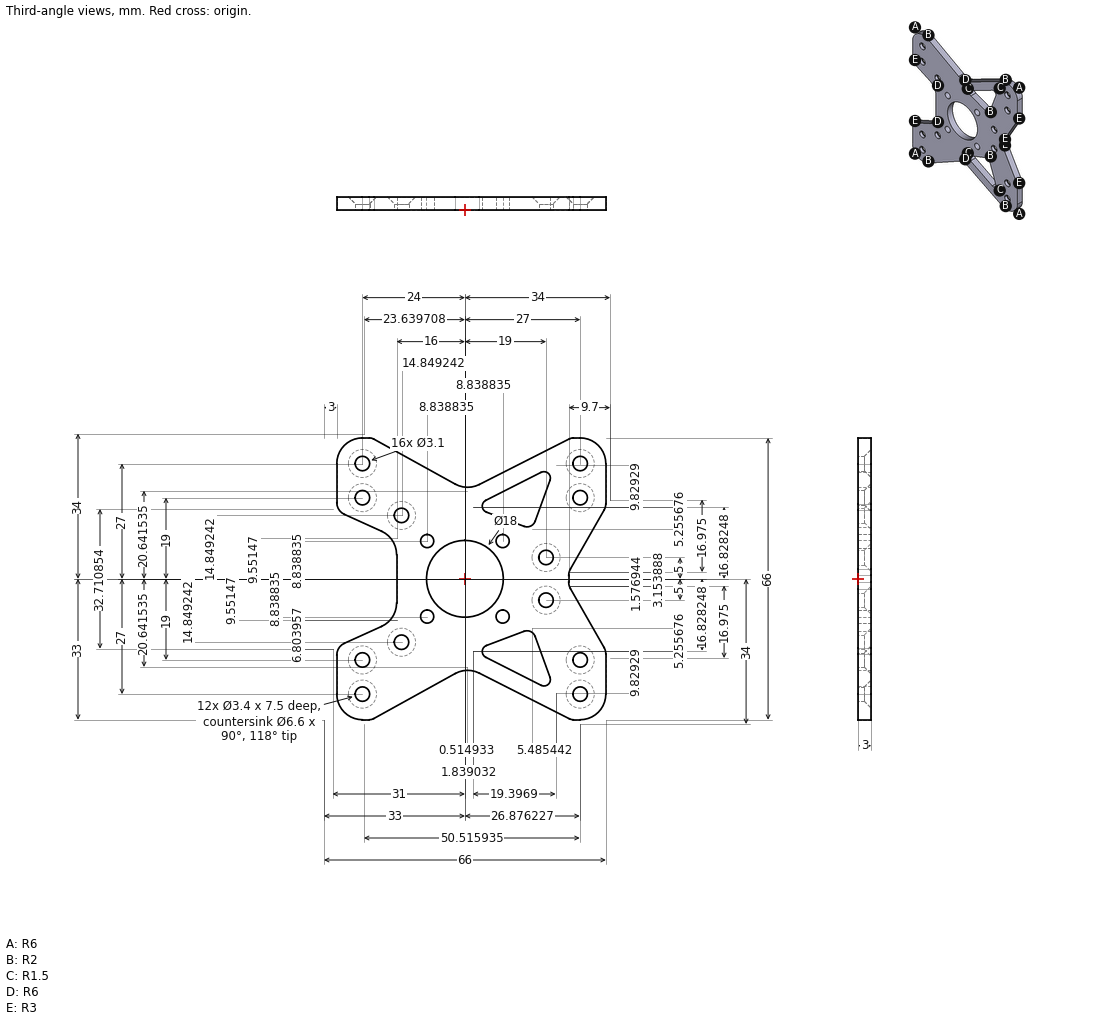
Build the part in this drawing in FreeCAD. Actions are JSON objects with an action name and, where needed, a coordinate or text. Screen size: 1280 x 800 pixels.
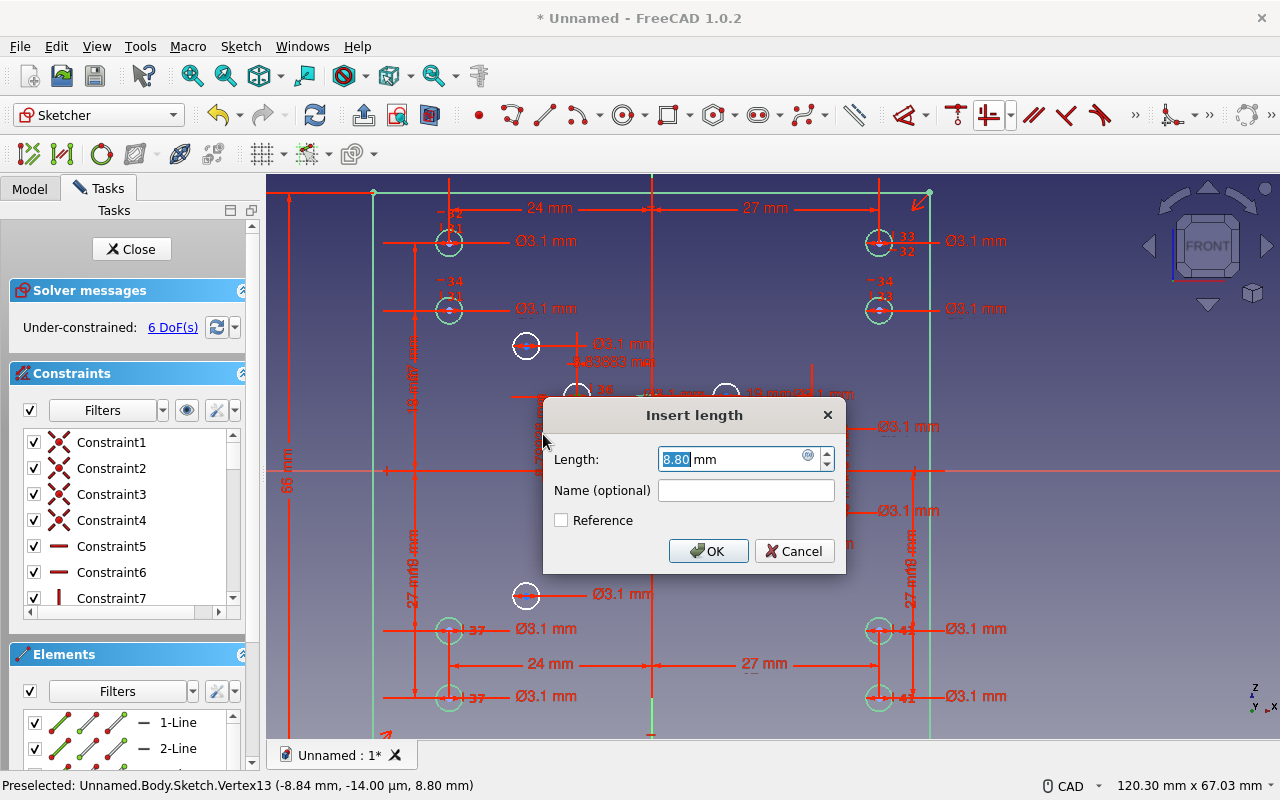
{"action": "type", "text": "8.838835"}
{"action": "key", "text": "Return"}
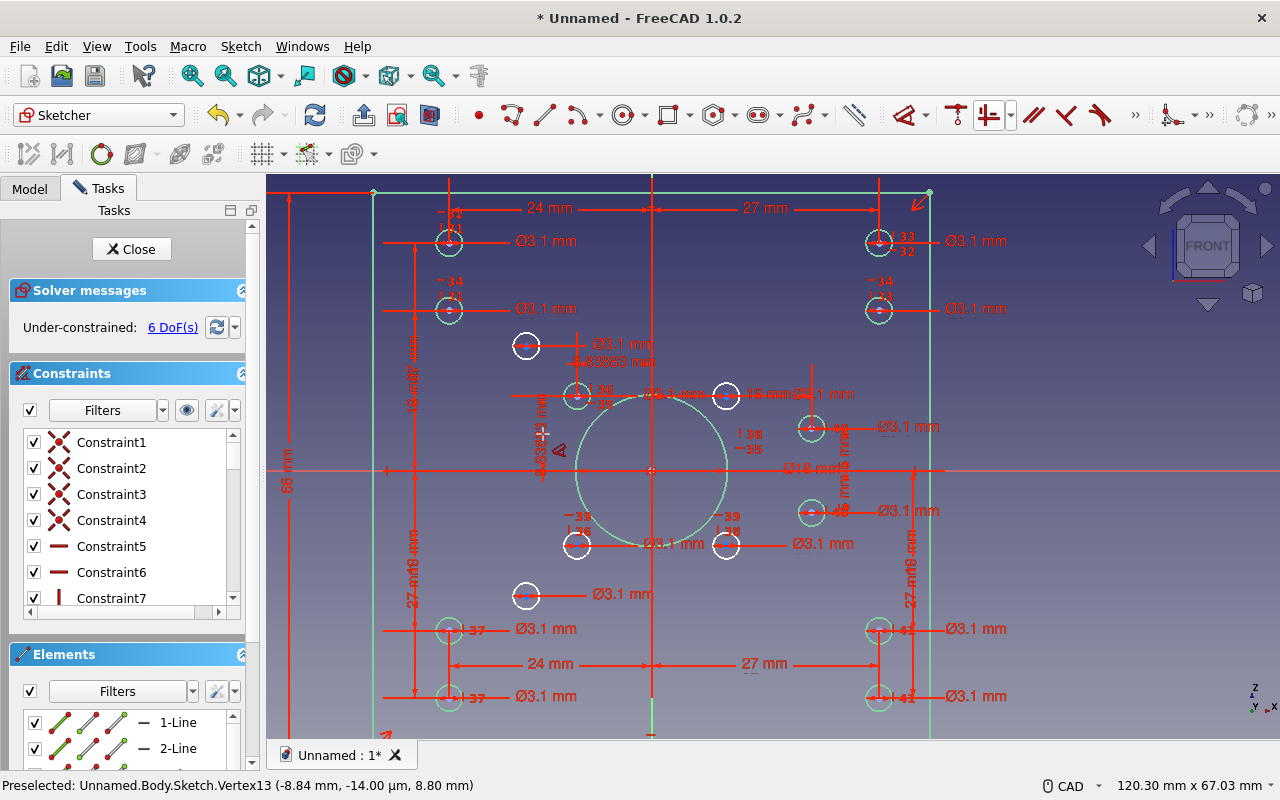
{"action": "left_click", "coordinate": [726, 396]}
{"action": "left_click", "coordinate": [689, 362]}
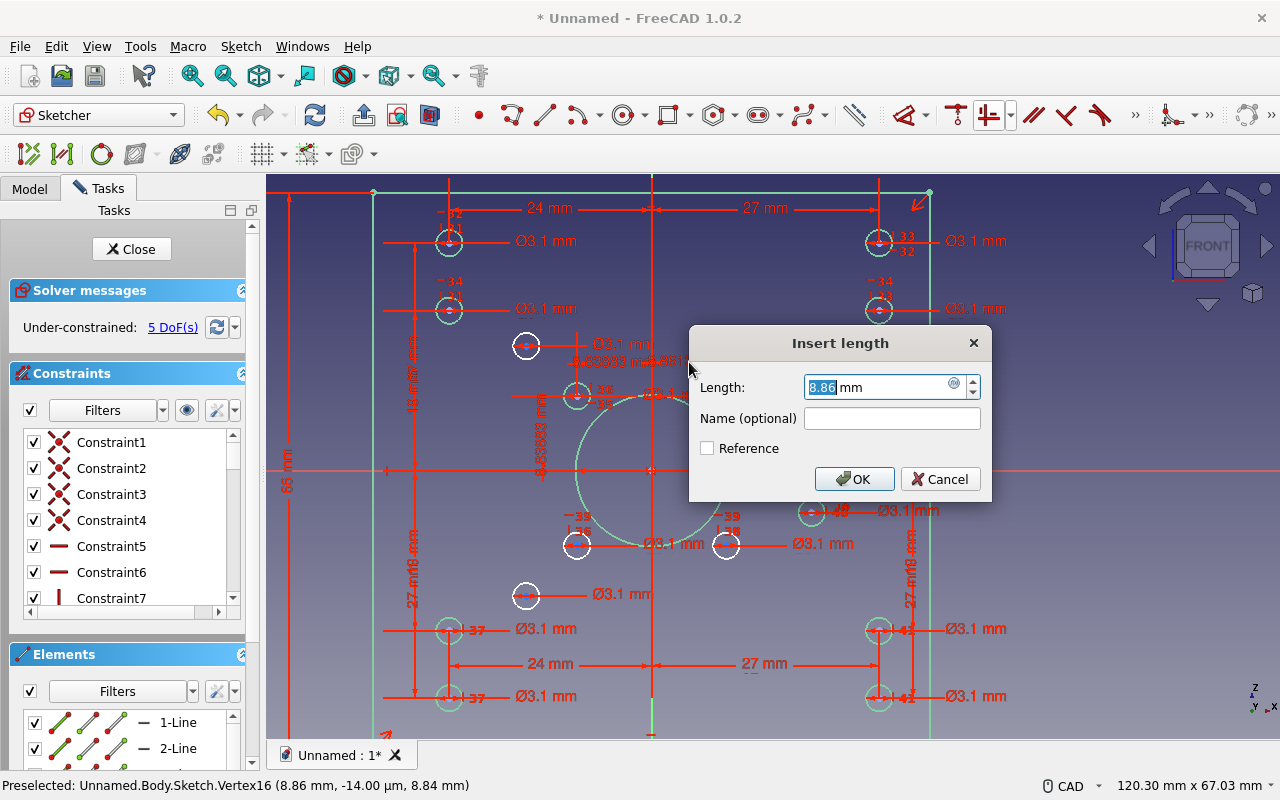
{"action": "type", "text": "8.838835"}
{"action": "key", "text": "Return"}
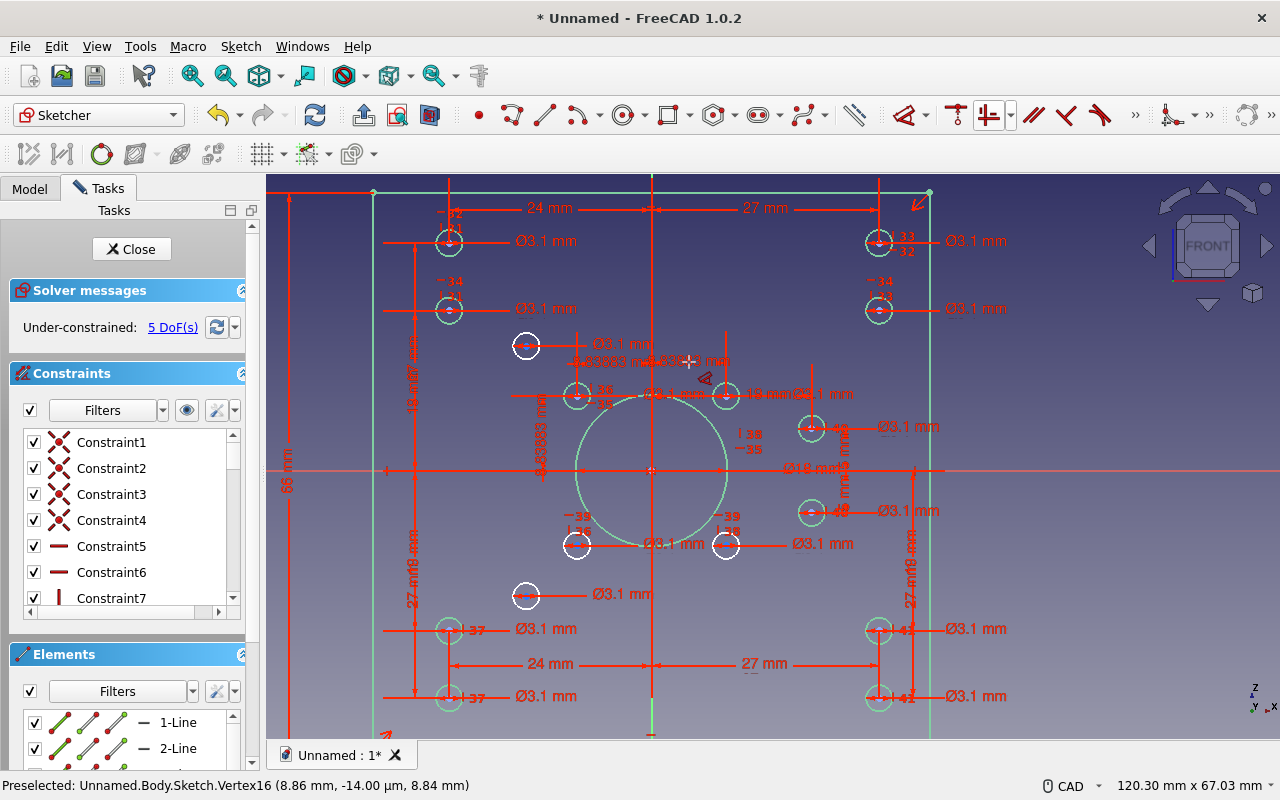
{"action": "left_click", "coordinate": [577, 546]}
{"action": "left_click", "coordinate": [543, 508]}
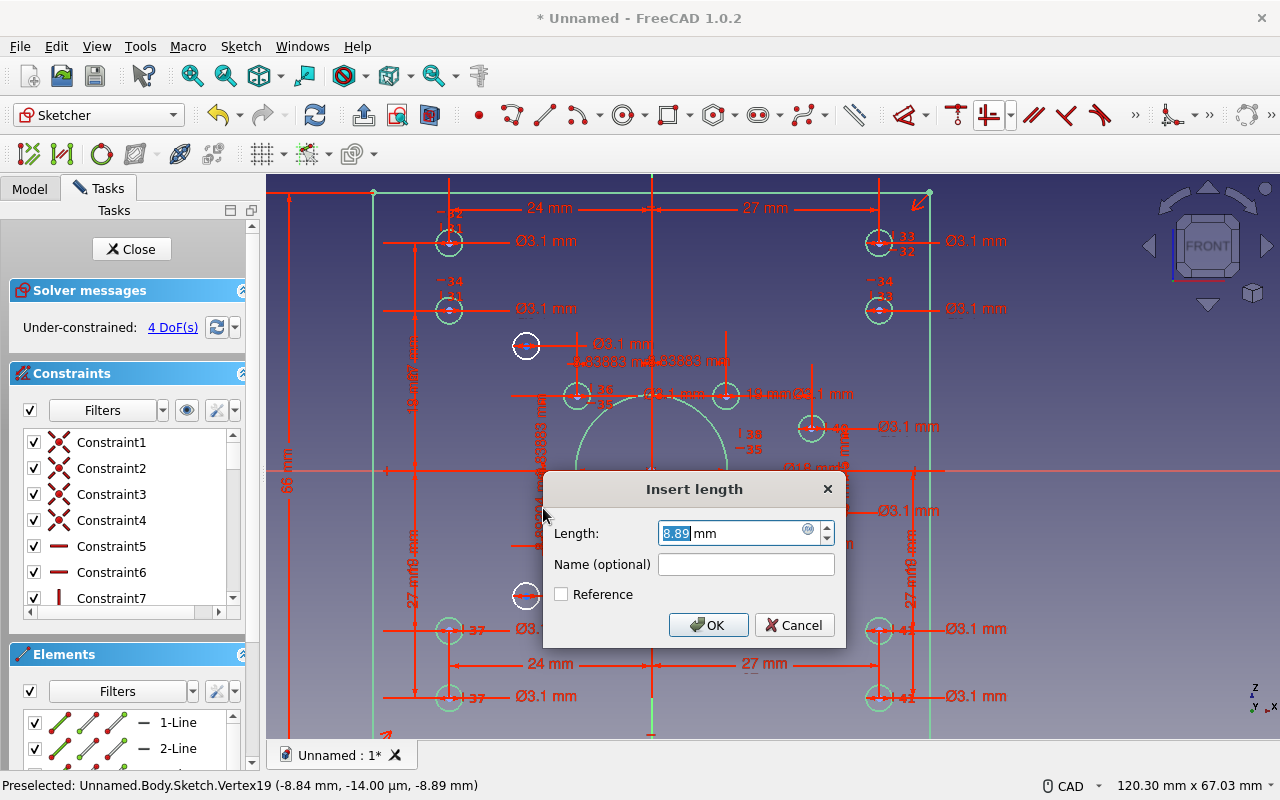
{"action": "type", "text": "8.838835"}
{"action": "key", "text": "Return"}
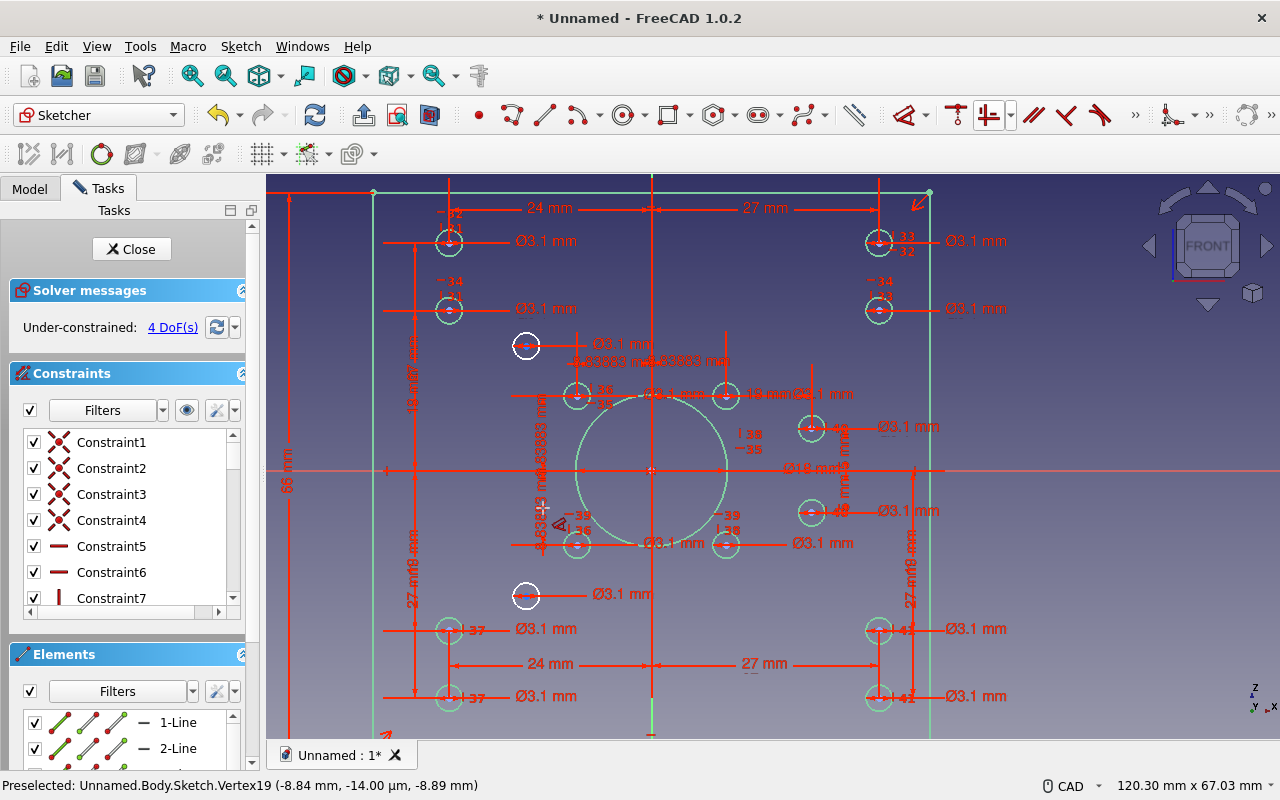
{"action": "left_click", "coordinate": [526, 346]}
{"action": "left_click", "coordinate": [589, 312]}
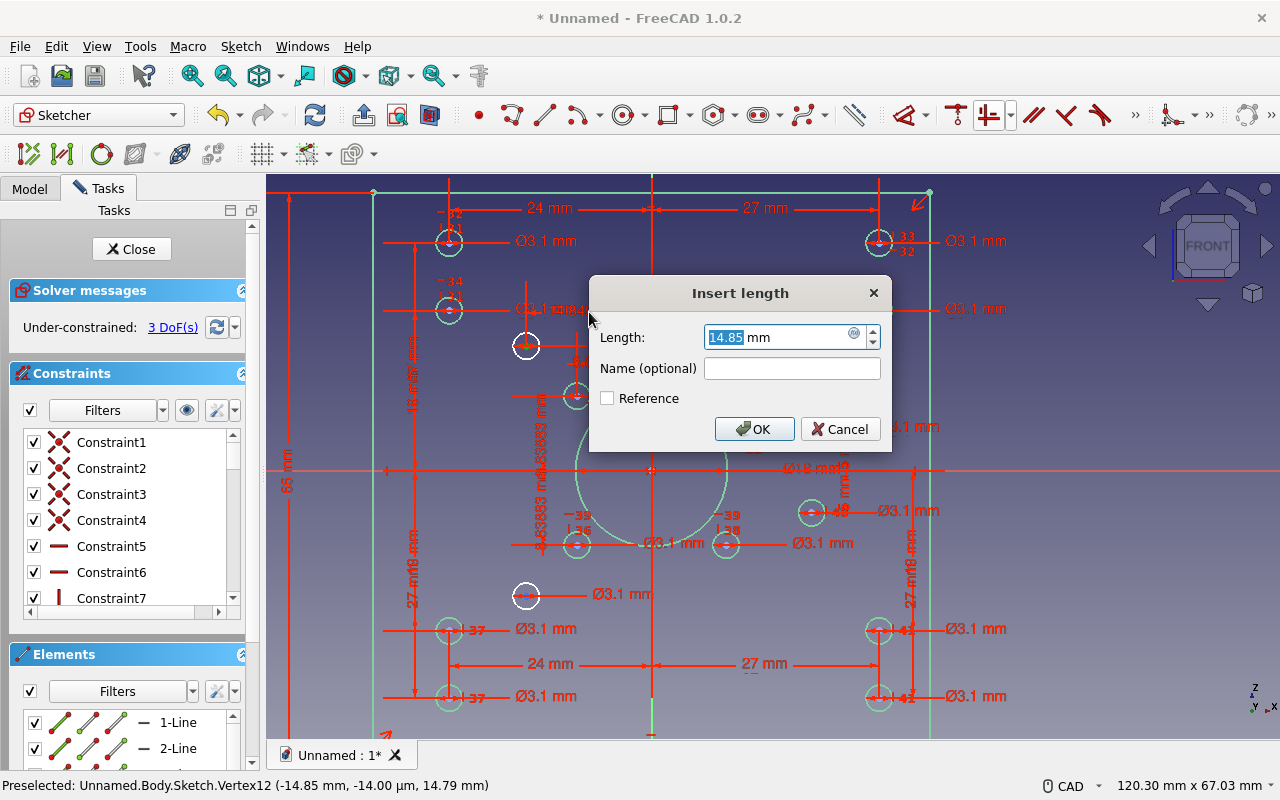
{"action": "type", "text": "14.849242"}
{"action": "key", "text": "Return"}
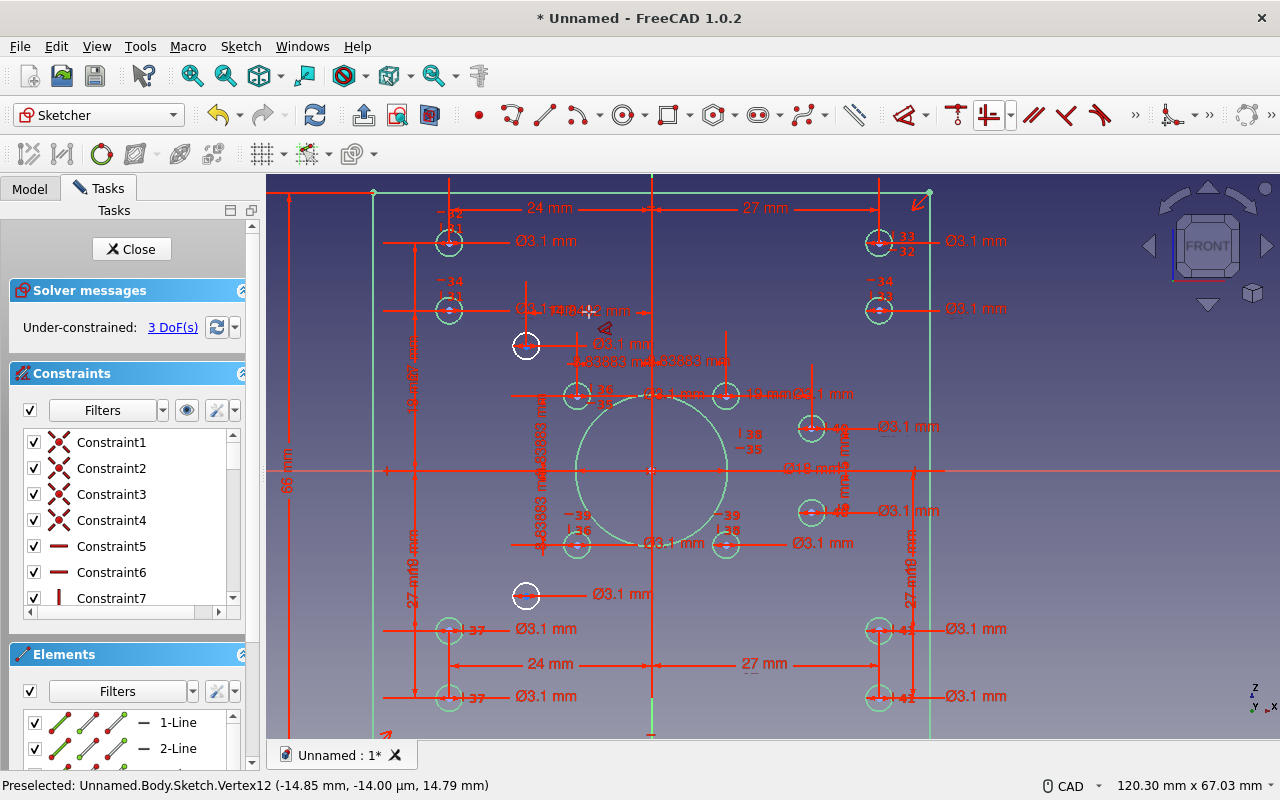
{"action": "left_click", "coordinate": [526, 346]}
{"action": "left_click", "coordinate": [492, 408]}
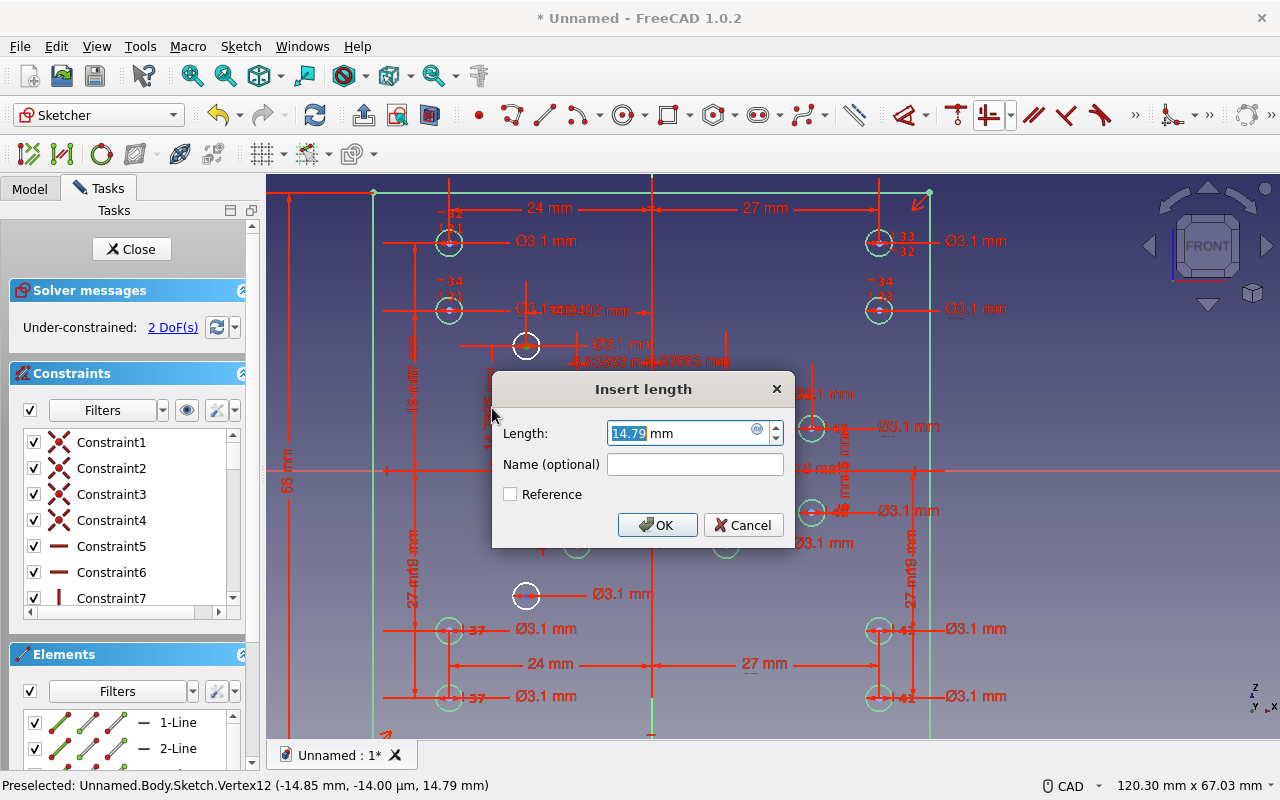
{"action": "type", "text": "14.849242"}
{"action": "key", "text": "Return"}